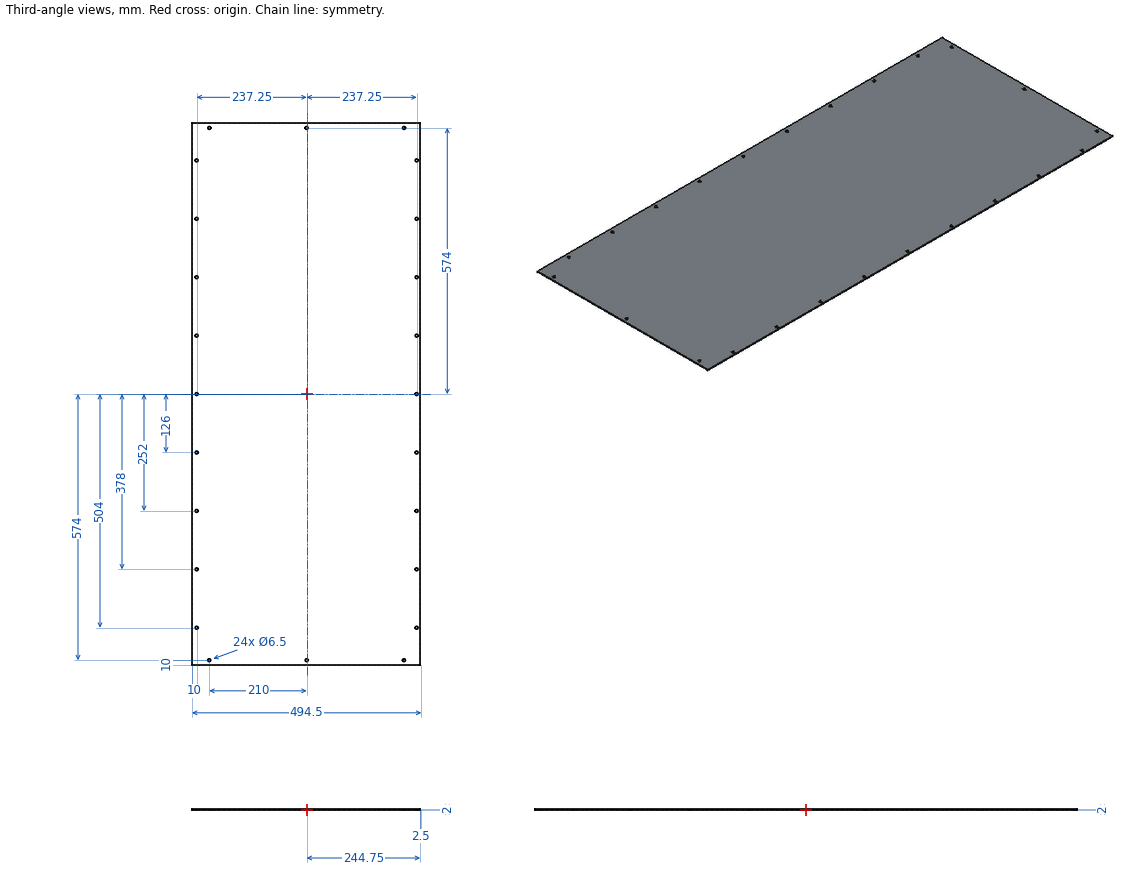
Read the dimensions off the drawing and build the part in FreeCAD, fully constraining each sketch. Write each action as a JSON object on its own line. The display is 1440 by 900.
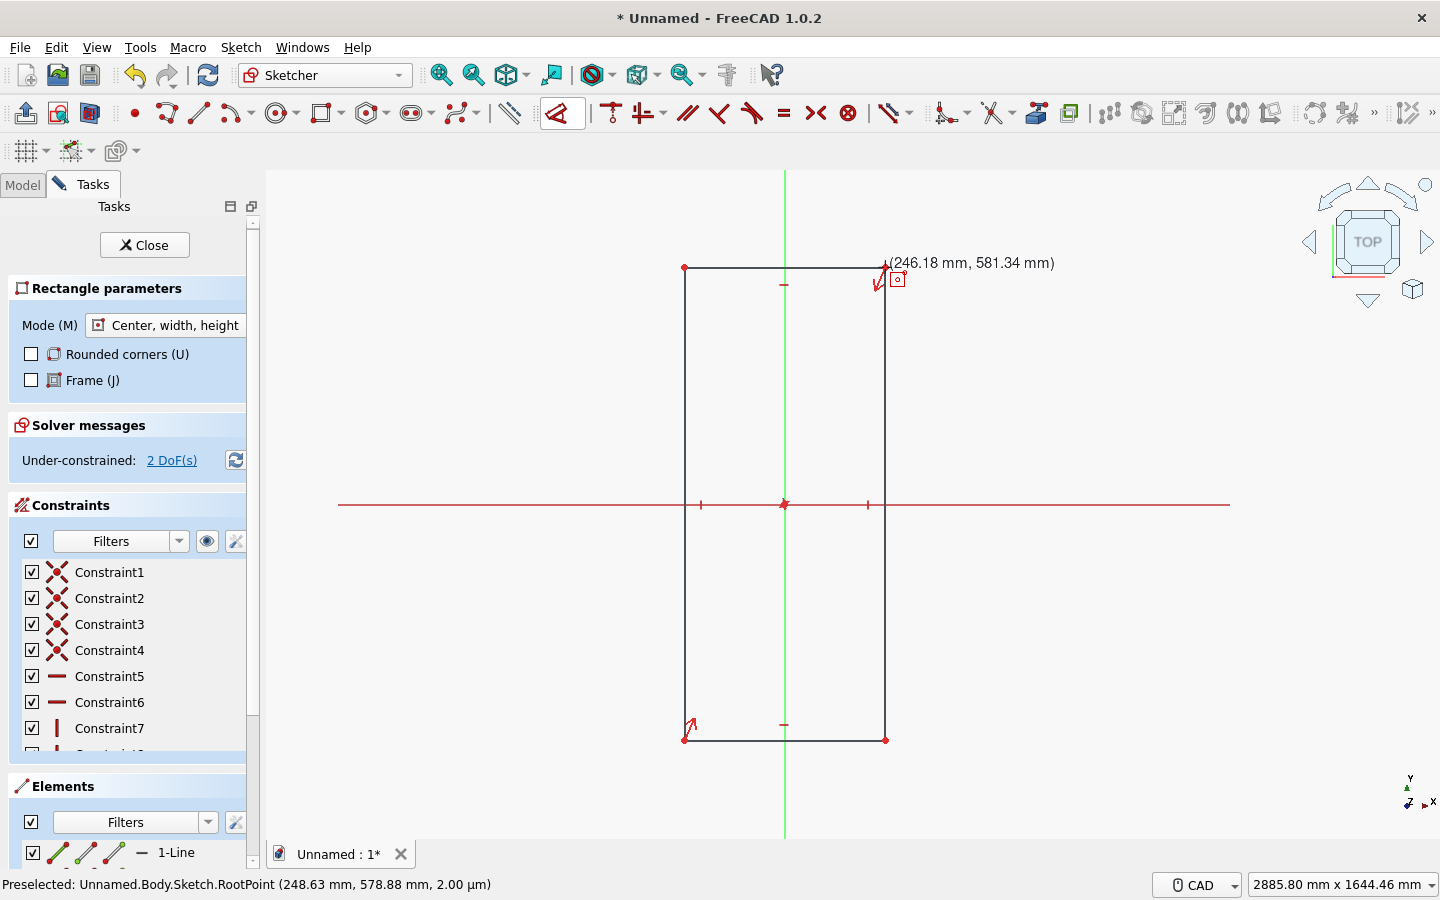
{"action": "left_click", "coordinate": [276, 114]}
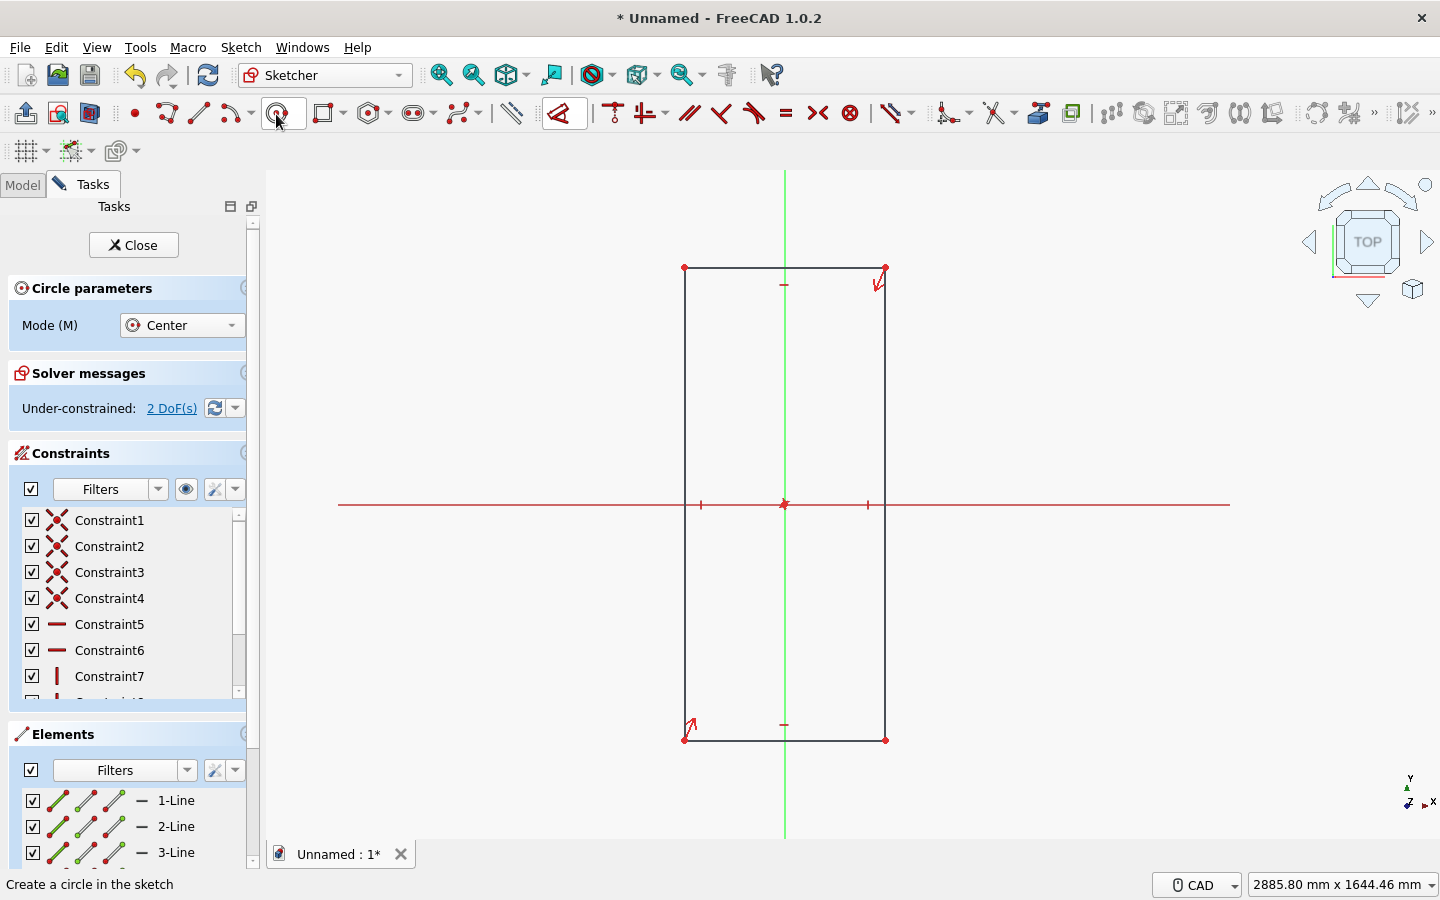
{"action": "scroll", "coordinate": [699, 738], "scroll_direction": "up", "scroll_amount": 15}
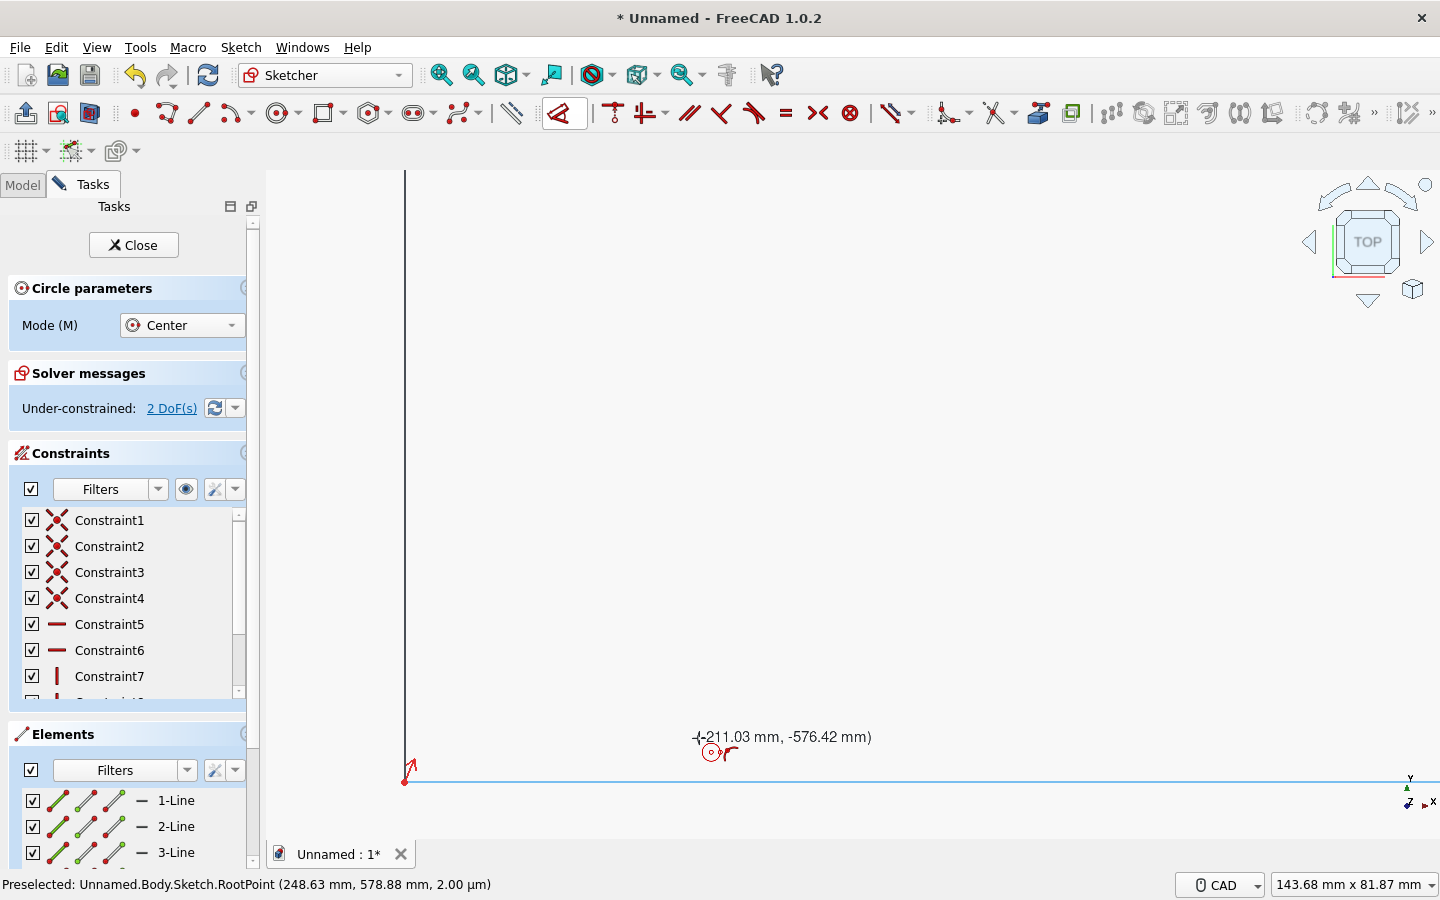
{"action": "scroll", "coordinate": [699, 739], "scroll_direction": "down", "scroll_amount": 15}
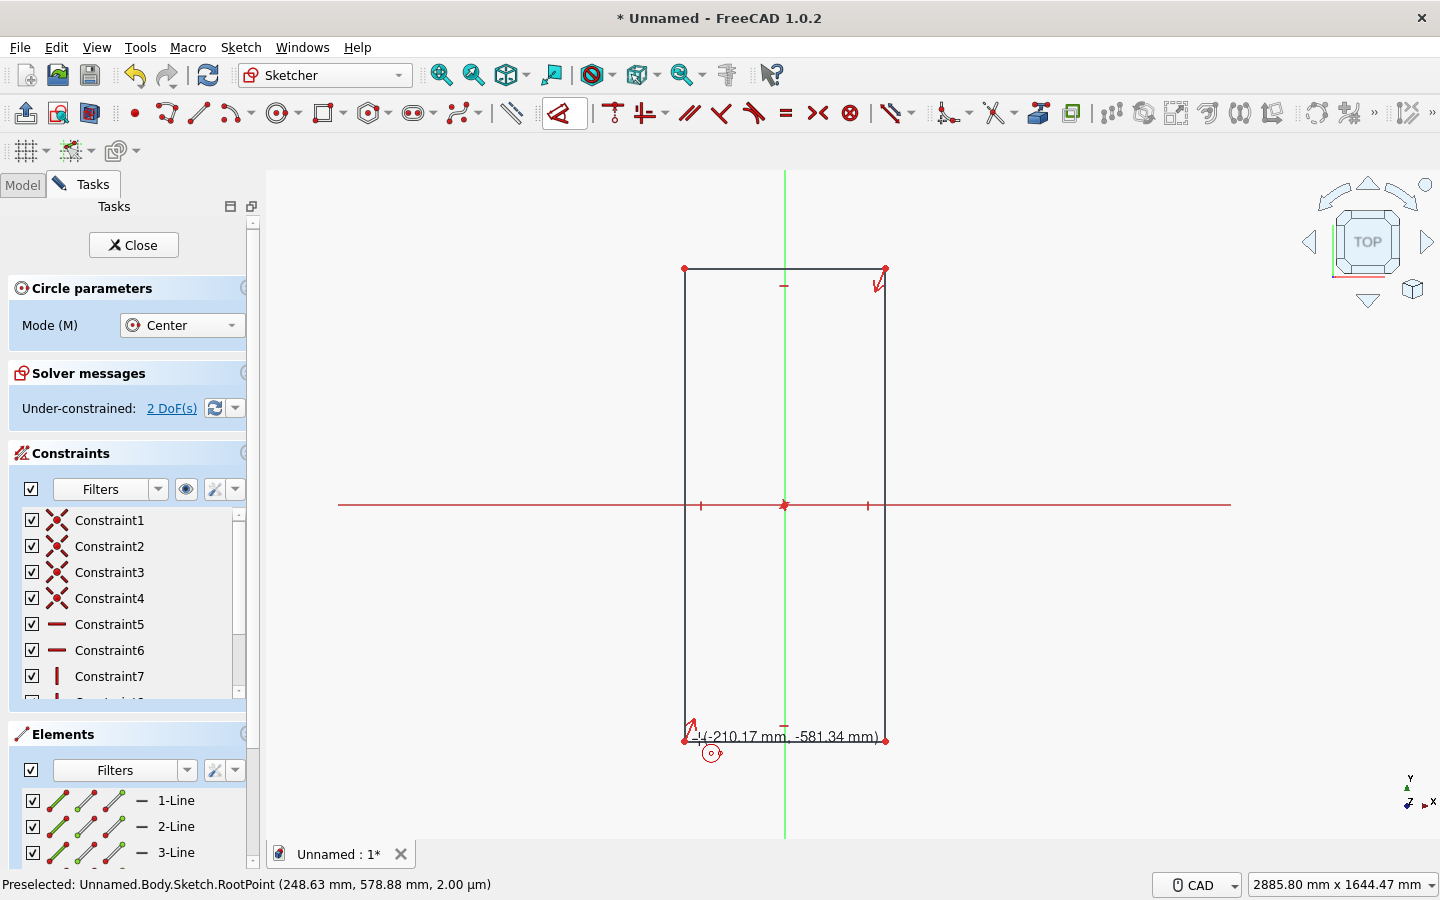
{"action": "scroll", "coordinate": [699, 739], "scroll_direction": "up", "scroll_amount": 7}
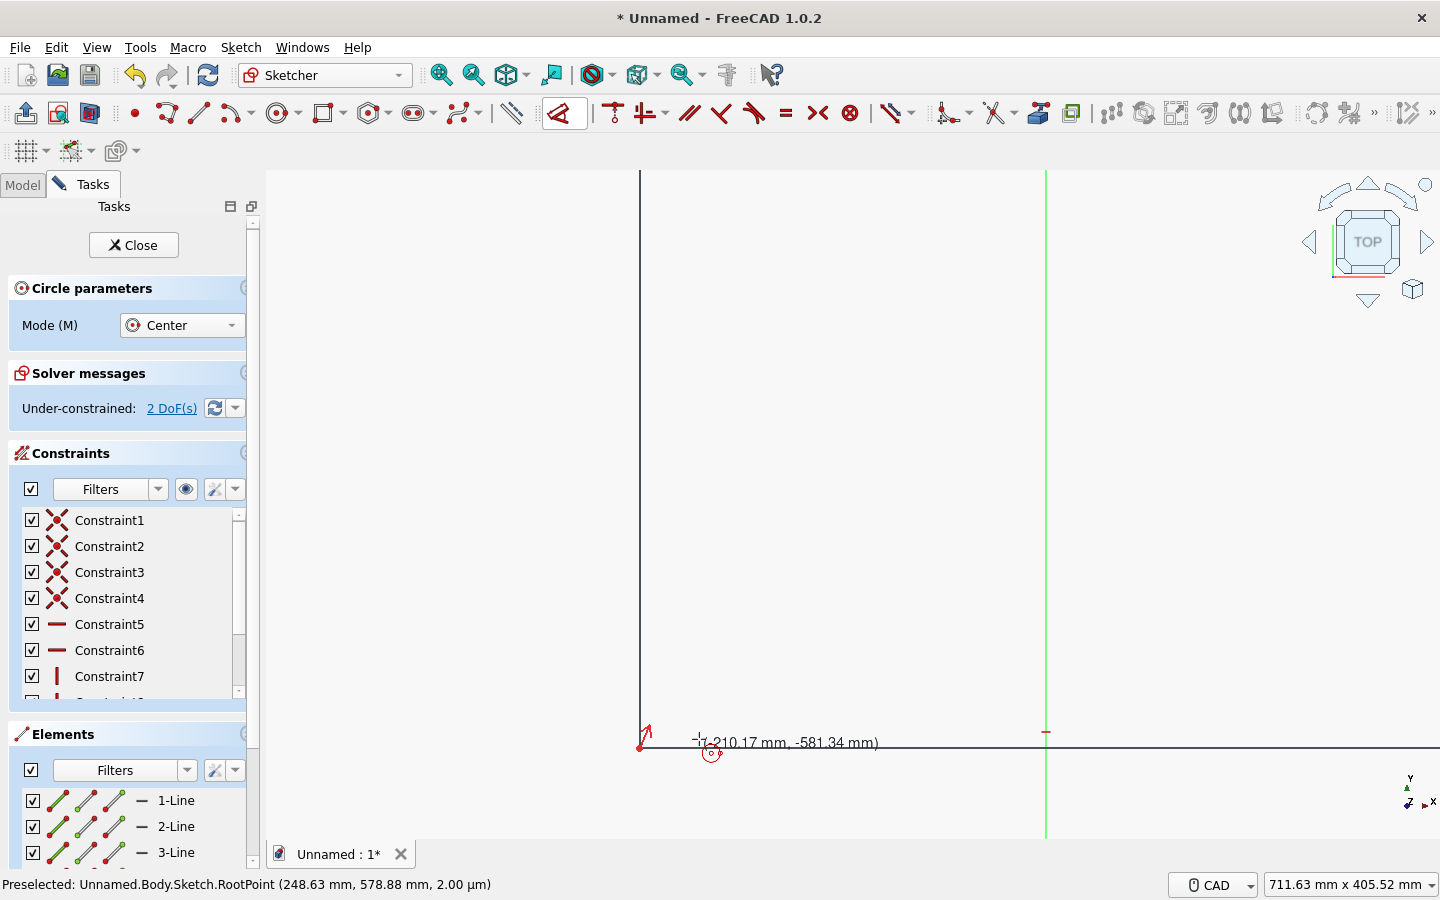
{"action": "left_click", "coordinate": [700, 736]}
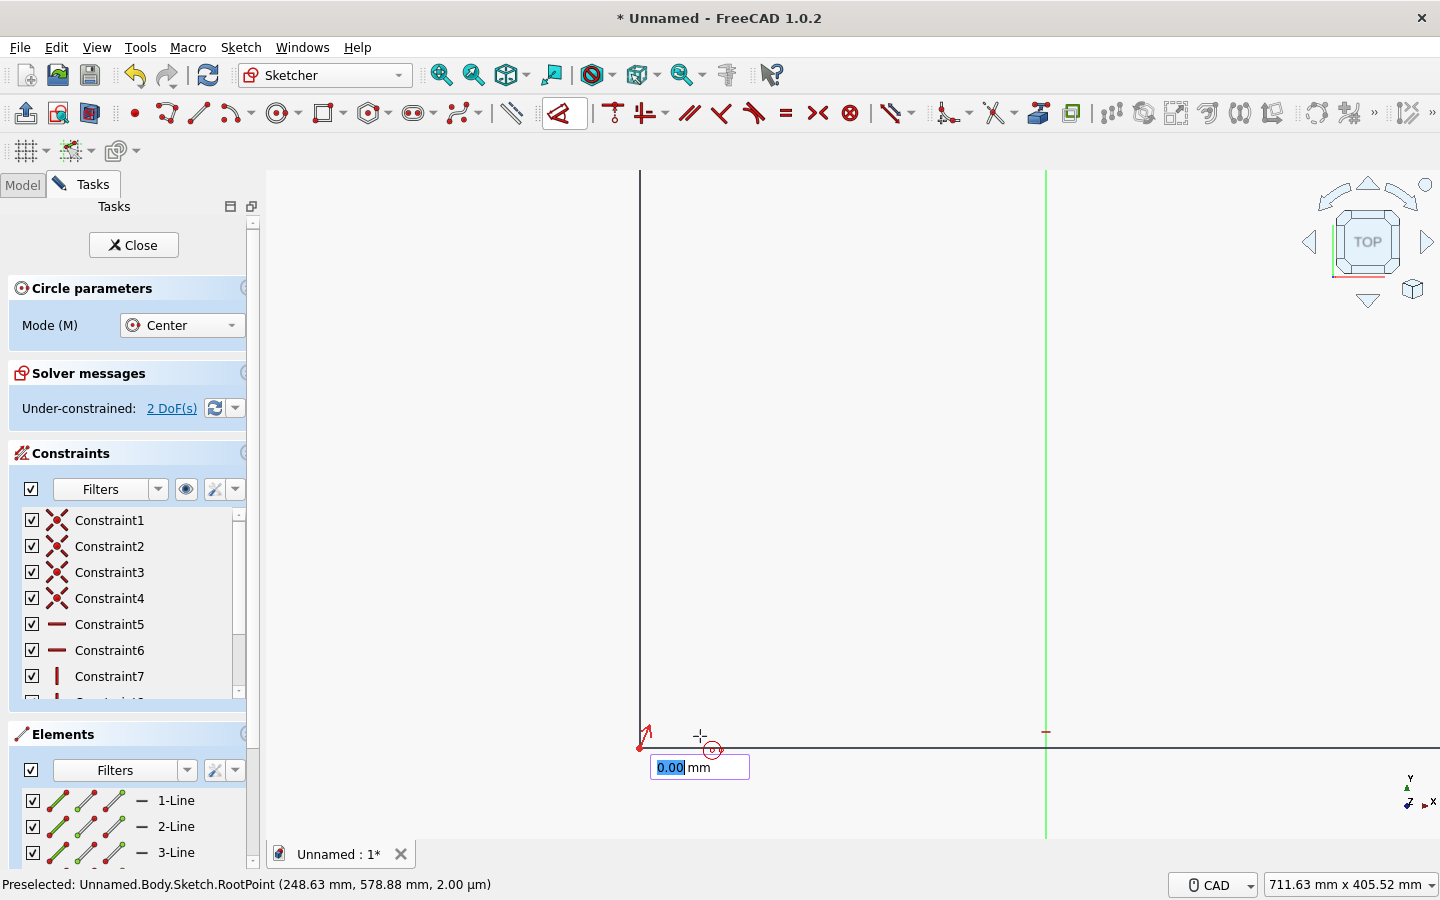
{"action": "scroll", "coordinate": [703, 732], "scroll_direction": "up", "scroll_amount": 6}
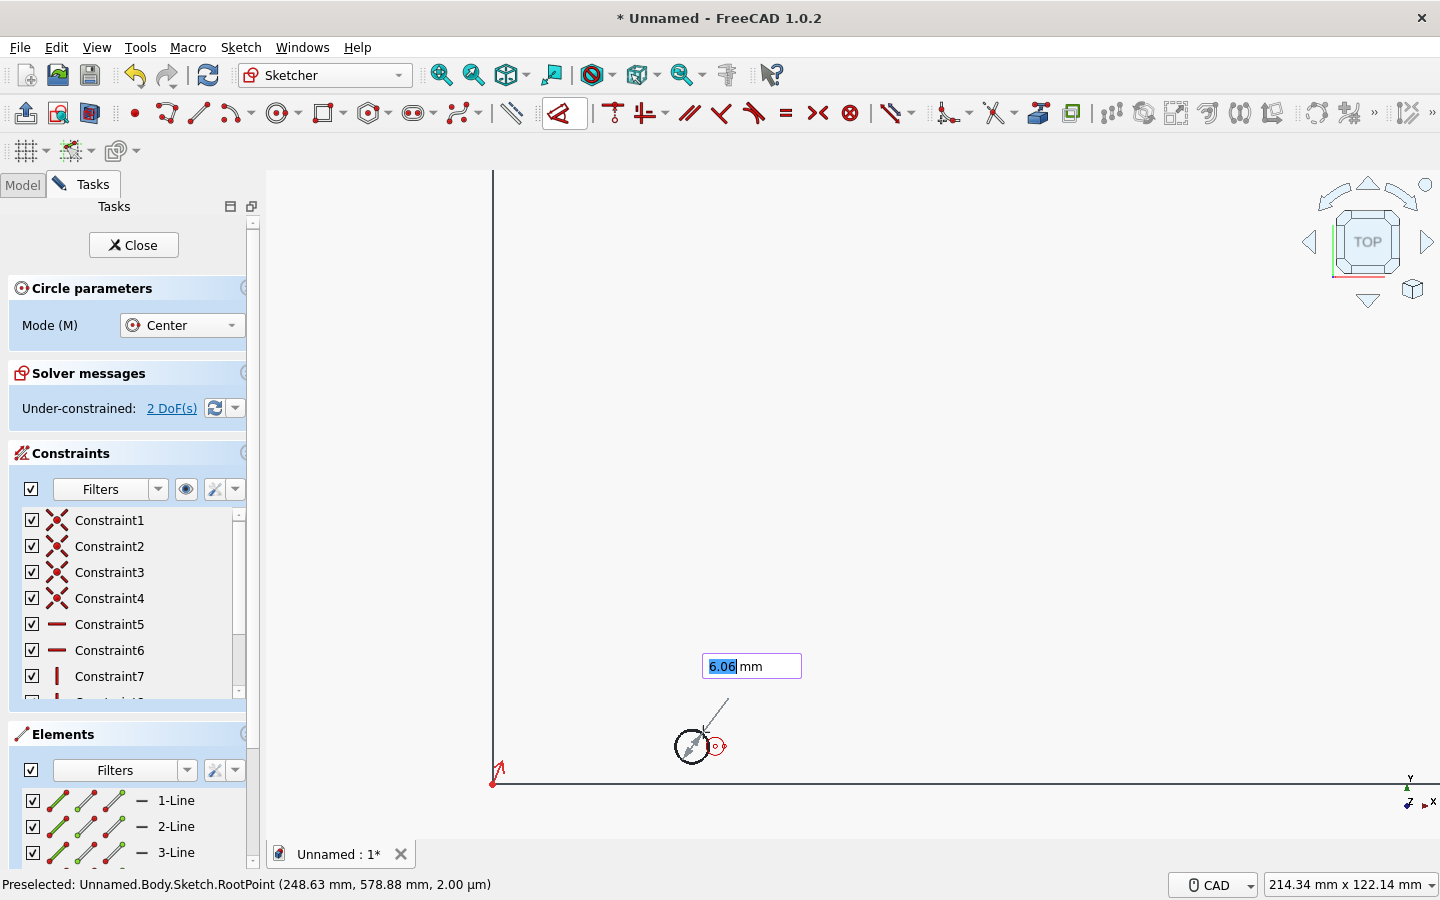
{"action": "left_click", "coordinate": [703, 732]}